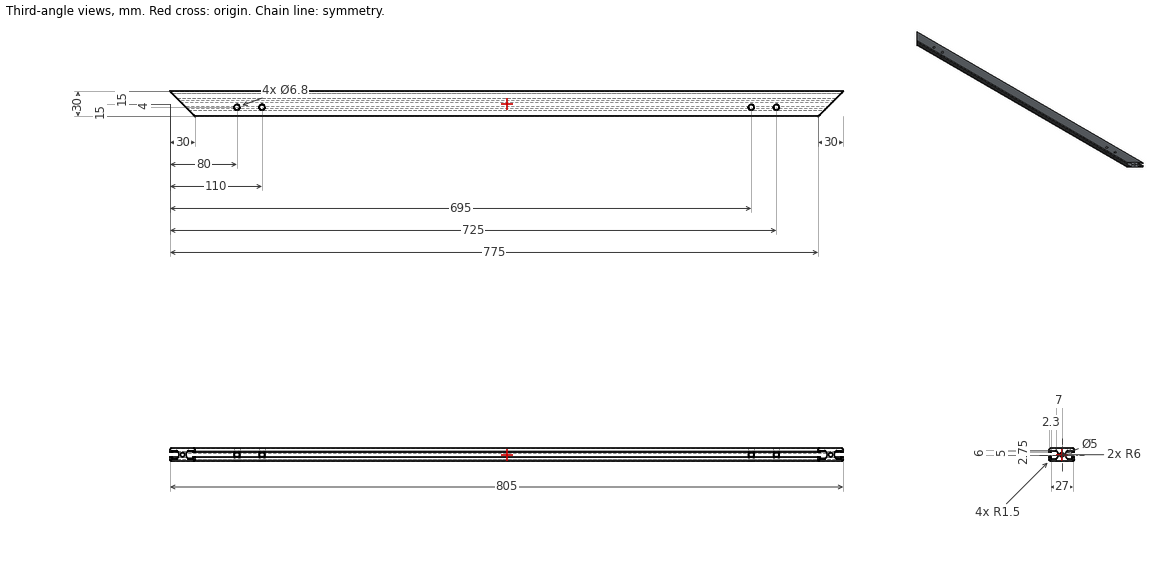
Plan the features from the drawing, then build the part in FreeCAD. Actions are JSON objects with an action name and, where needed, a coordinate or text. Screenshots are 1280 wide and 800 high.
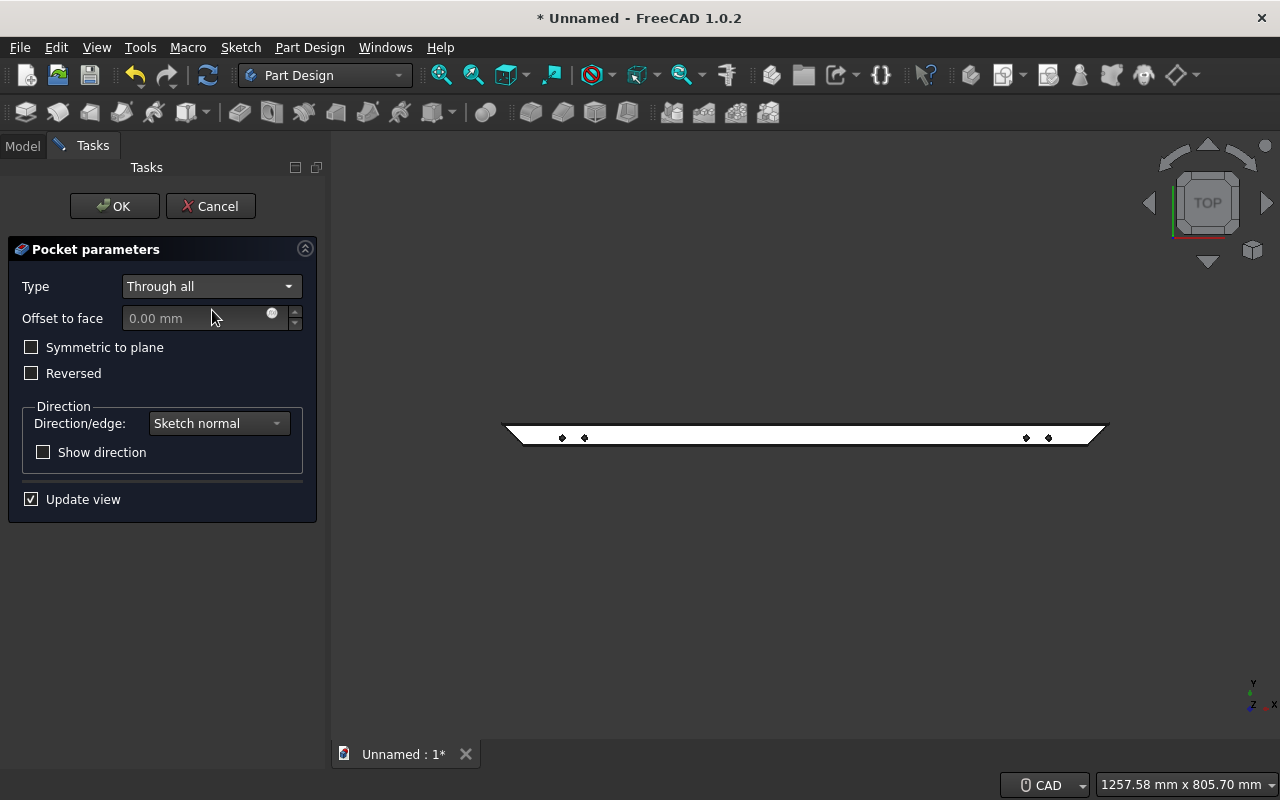
{"action": "left_click", "coordinate": [115, 206]}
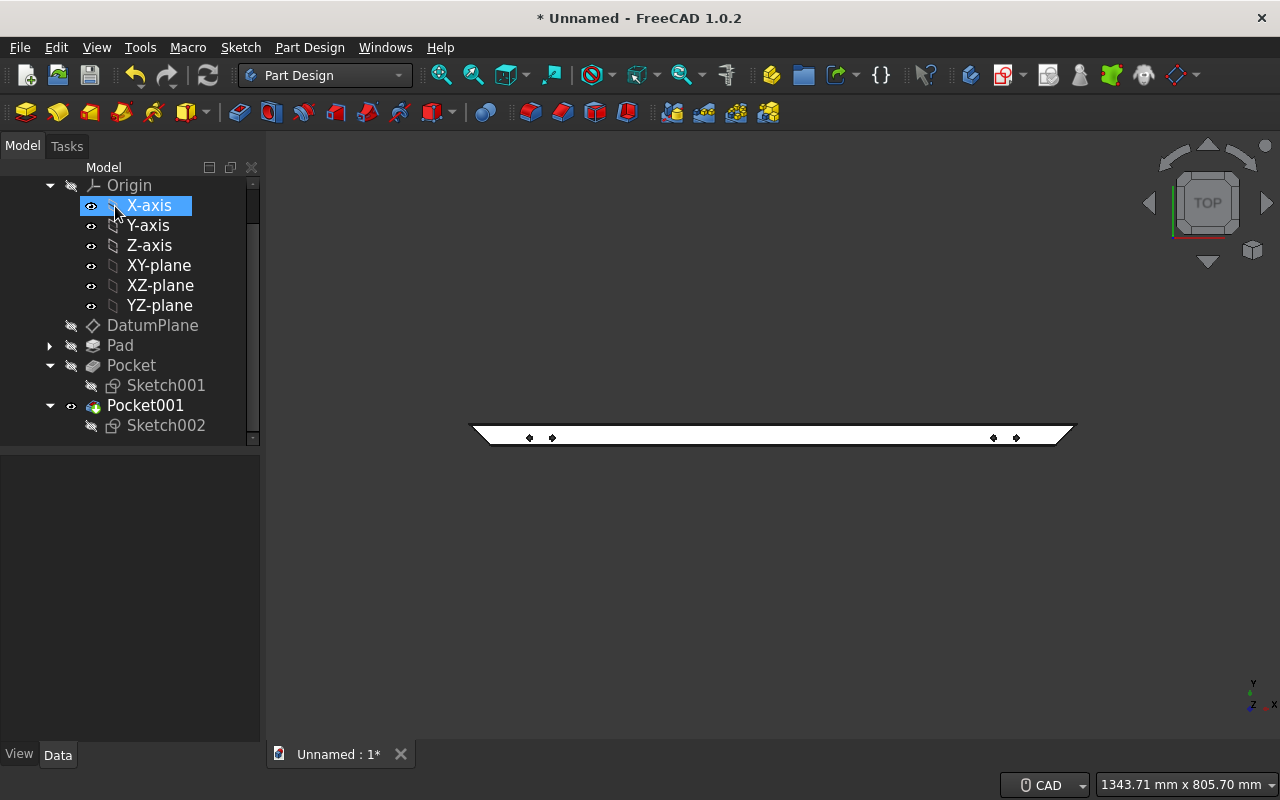
{"action": "key", "text": "0"}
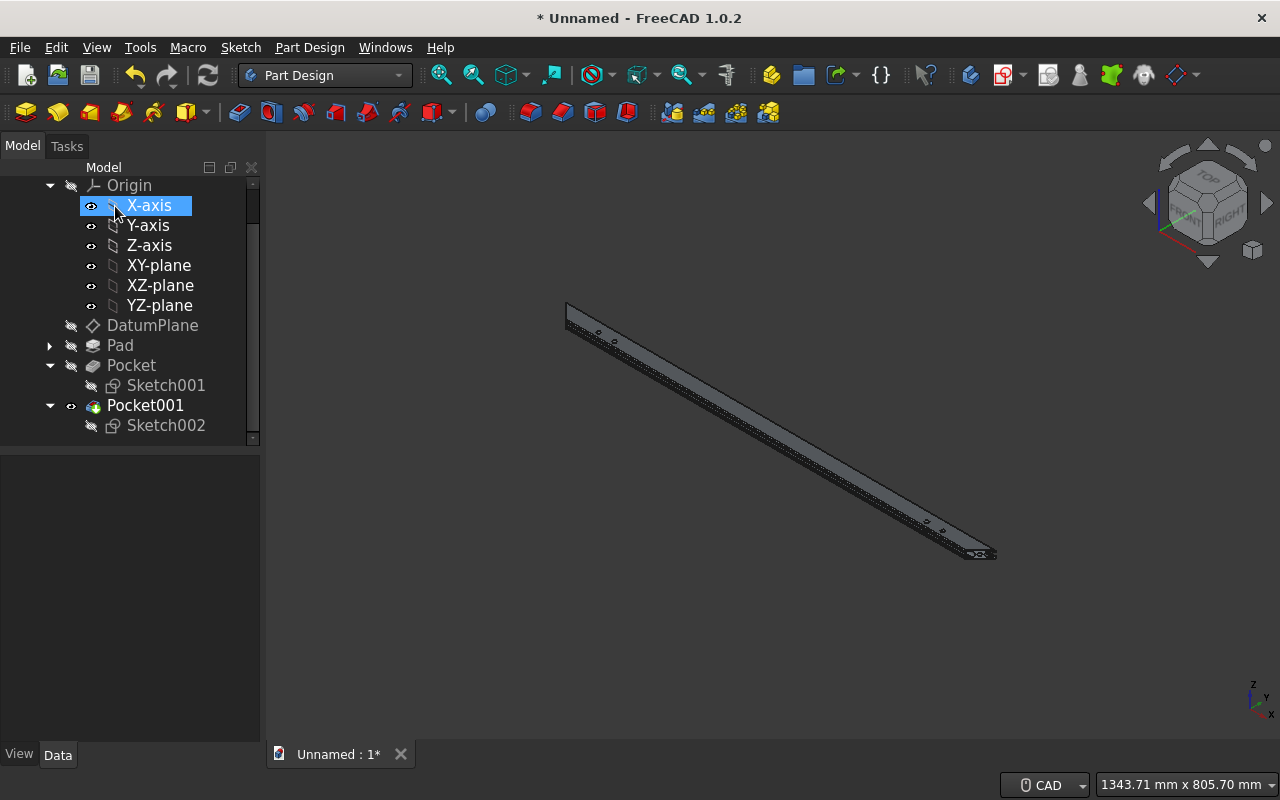
{"action": "left_click", "coordinate": [442, 76]}